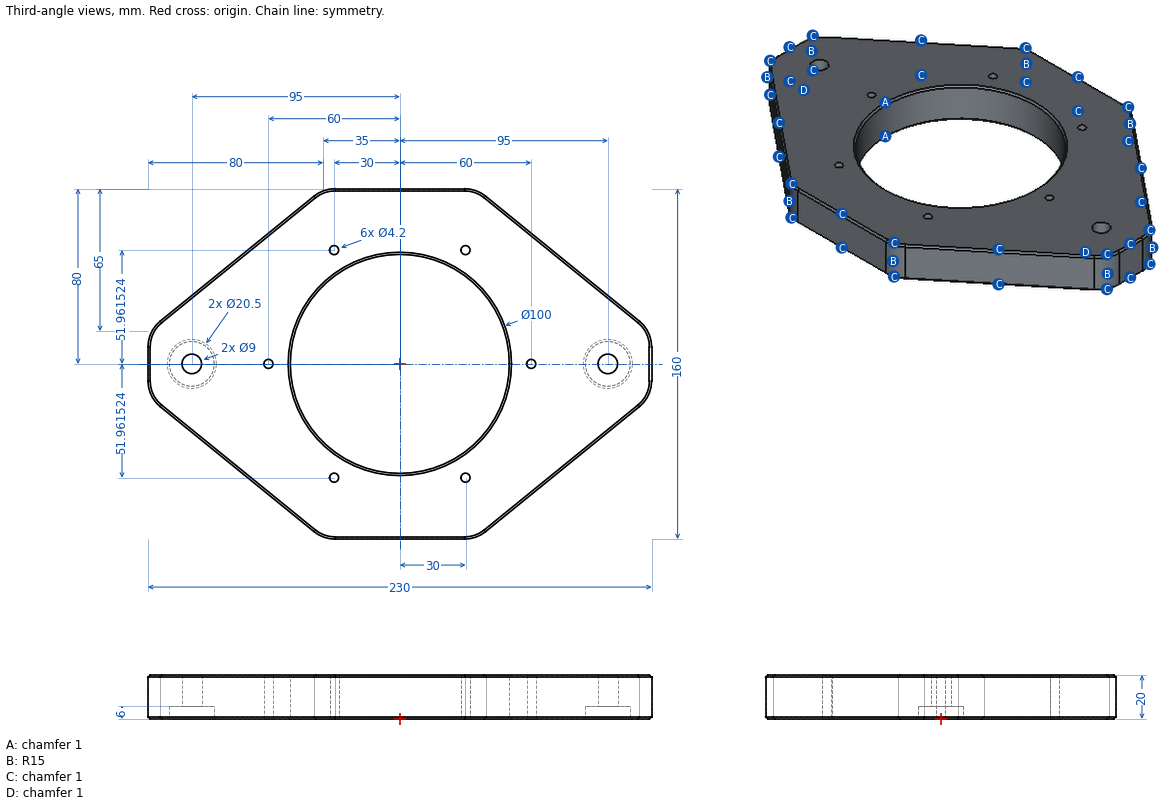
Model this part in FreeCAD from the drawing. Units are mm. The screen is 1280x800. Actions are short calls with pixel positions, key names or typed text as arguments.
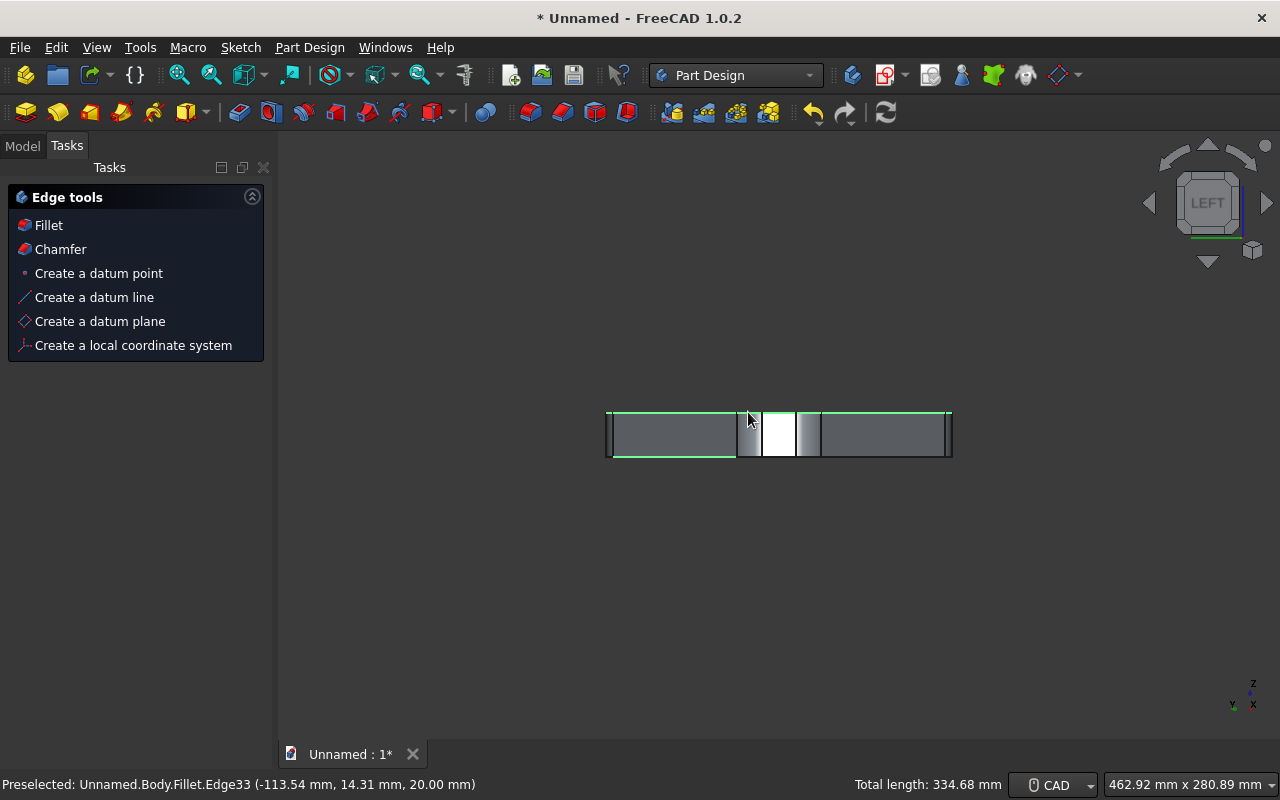
click(779, 456, ctrl)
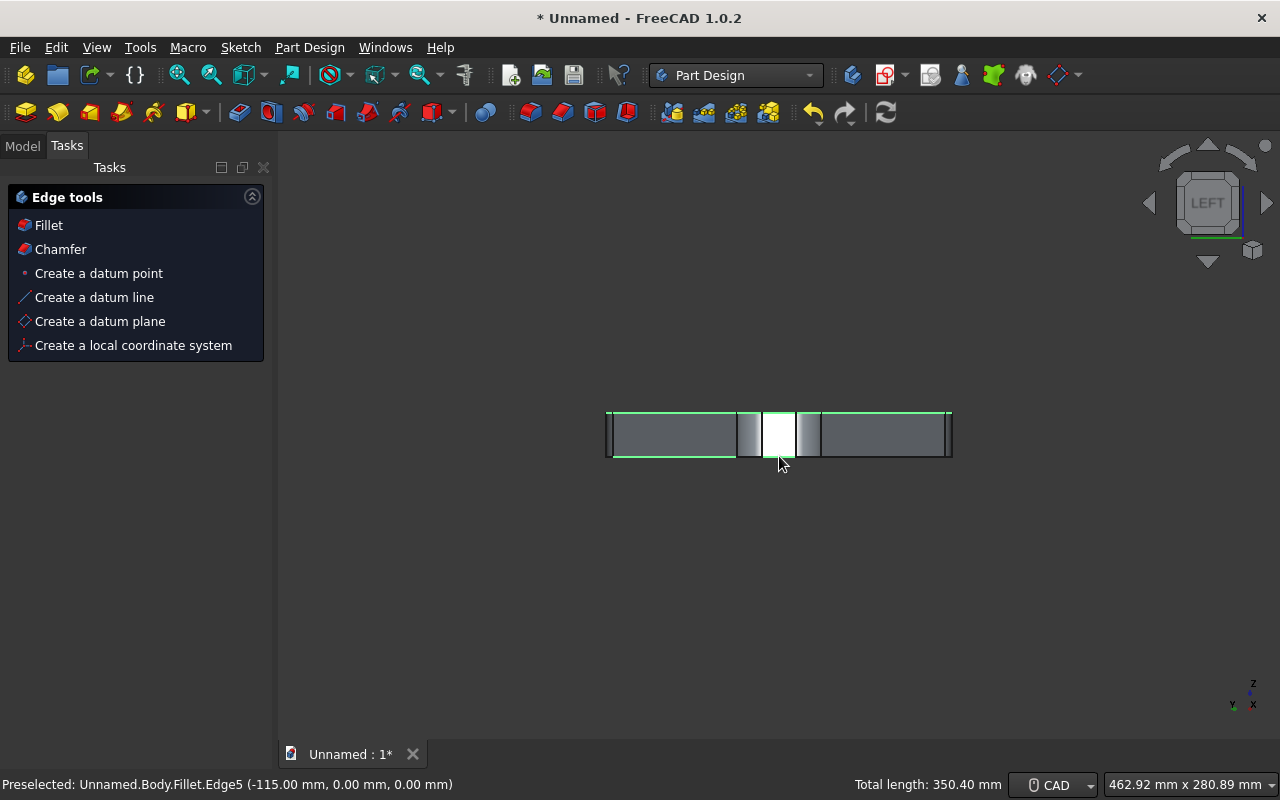
click(883, 456, ctrl)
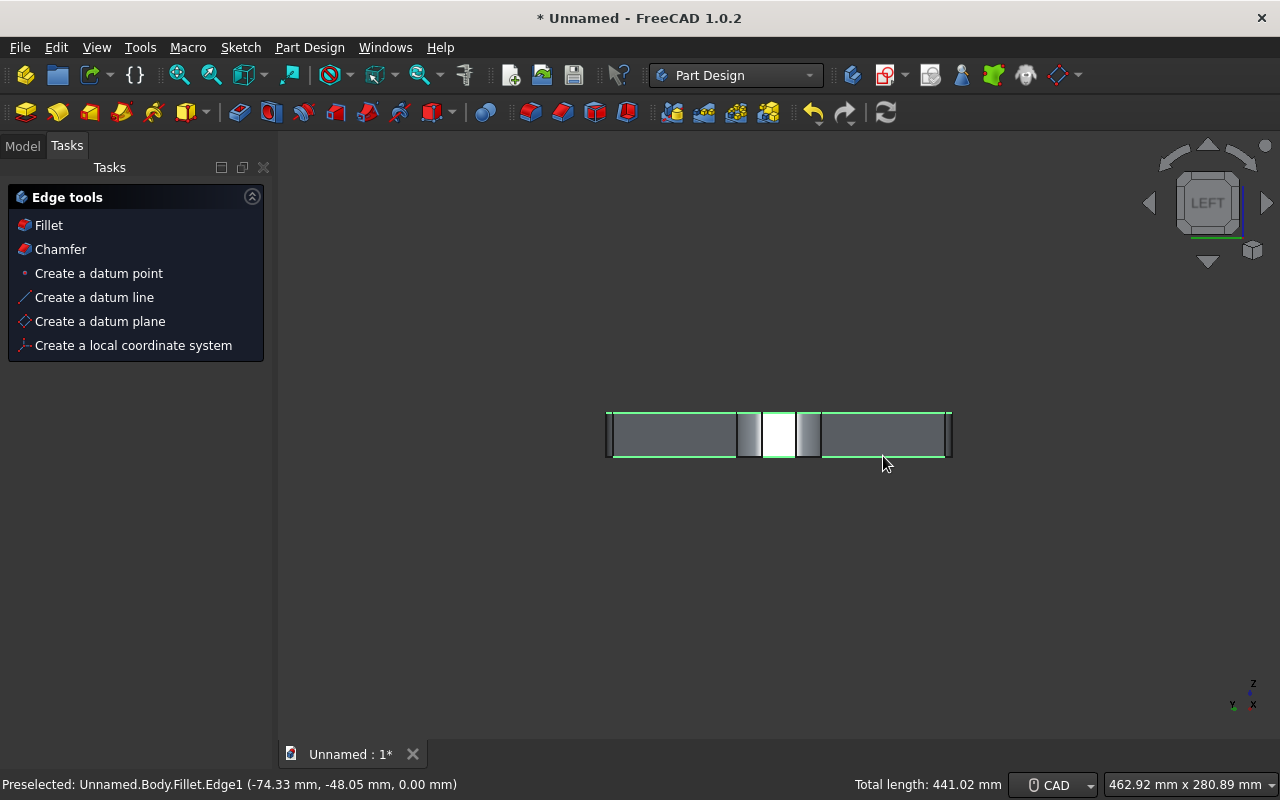
click(810, 456, ctrl)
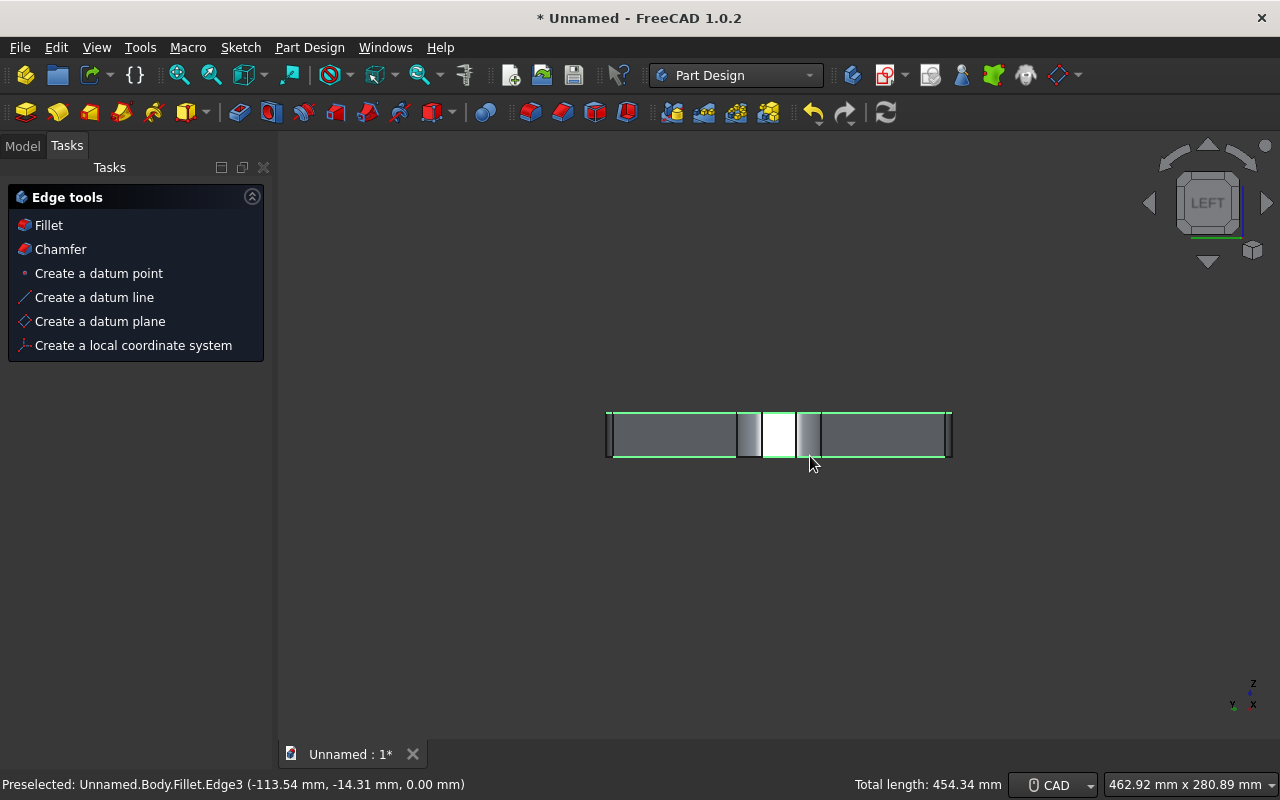
click(951, 456, ctrl)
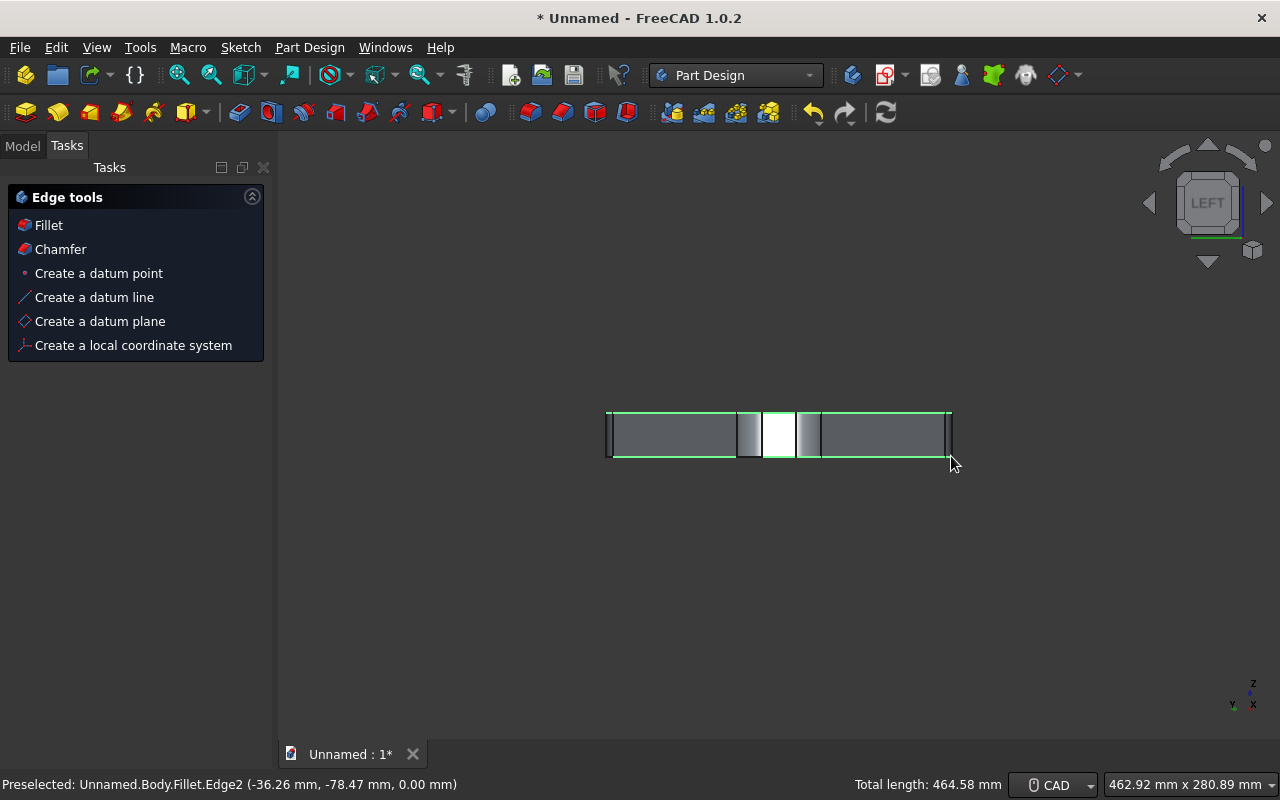
click(607, 456, ctrl)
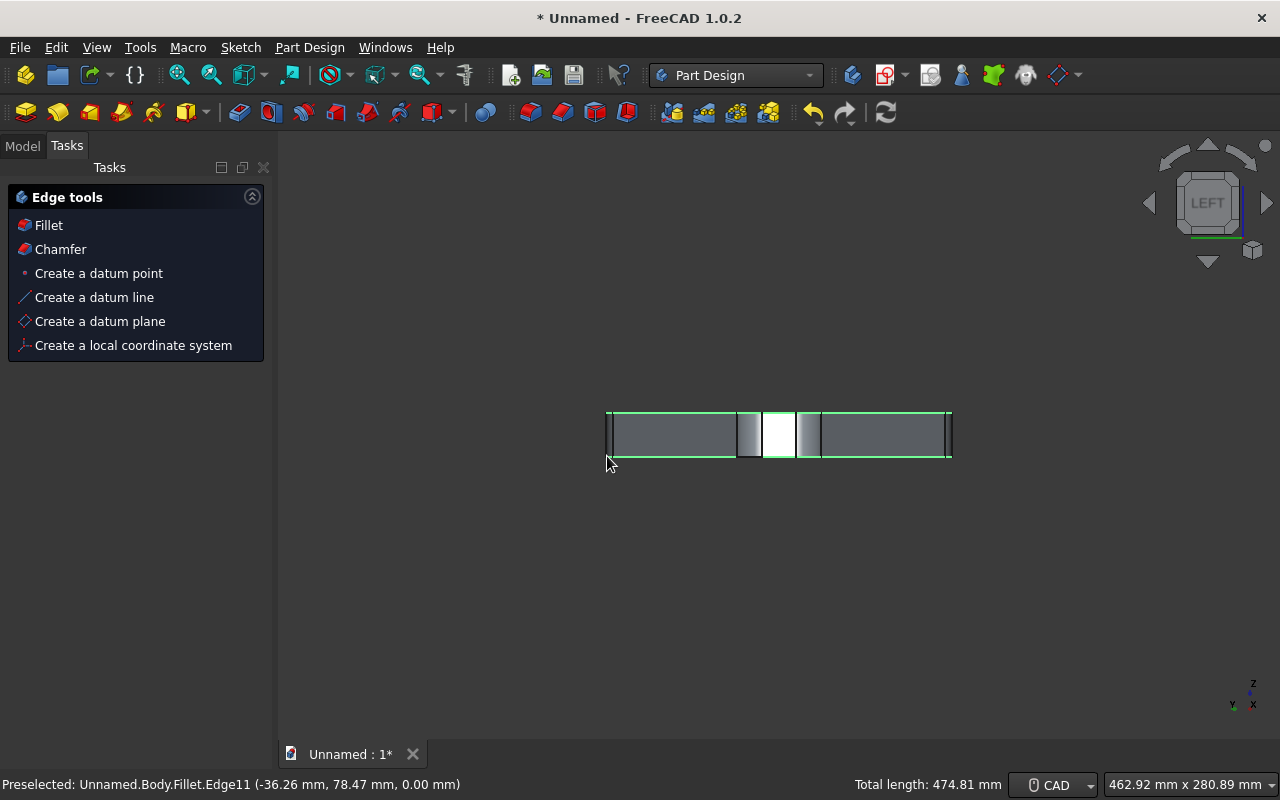
click(748, 456, ctrl)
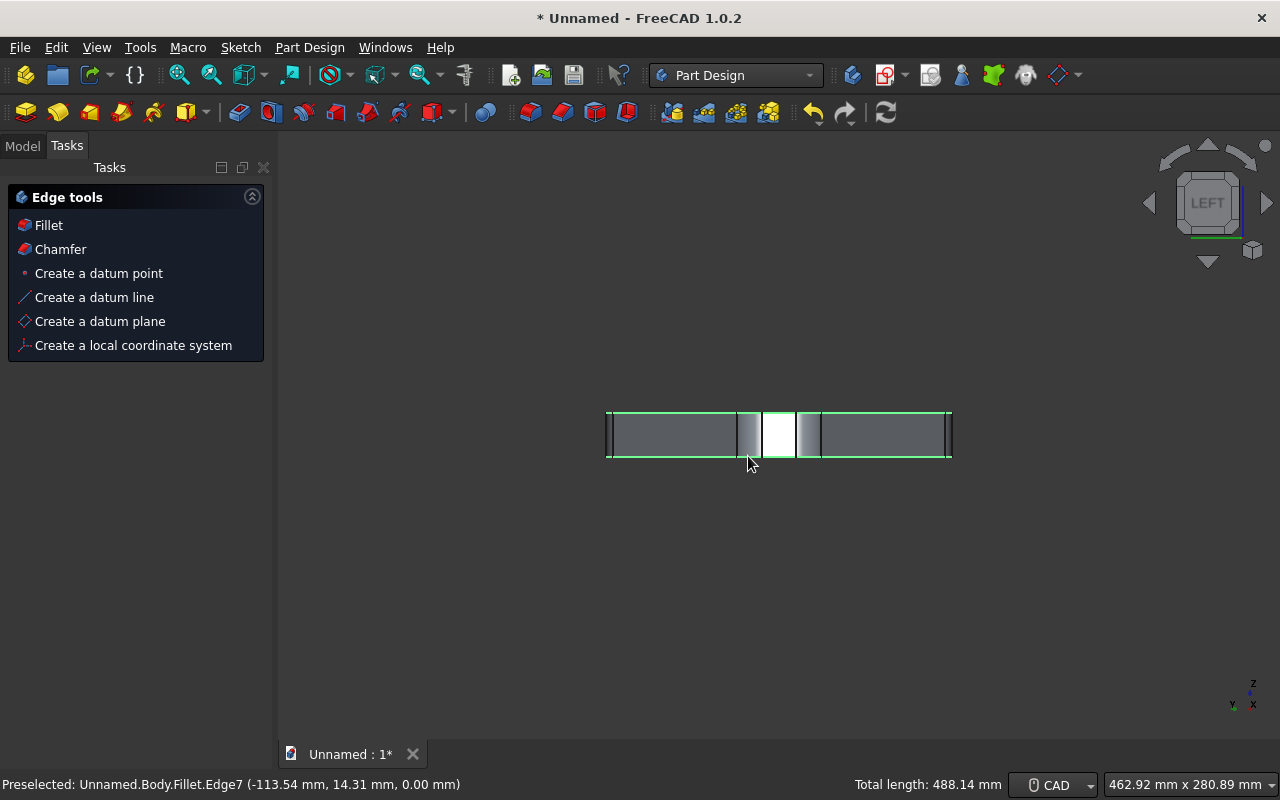
key(0)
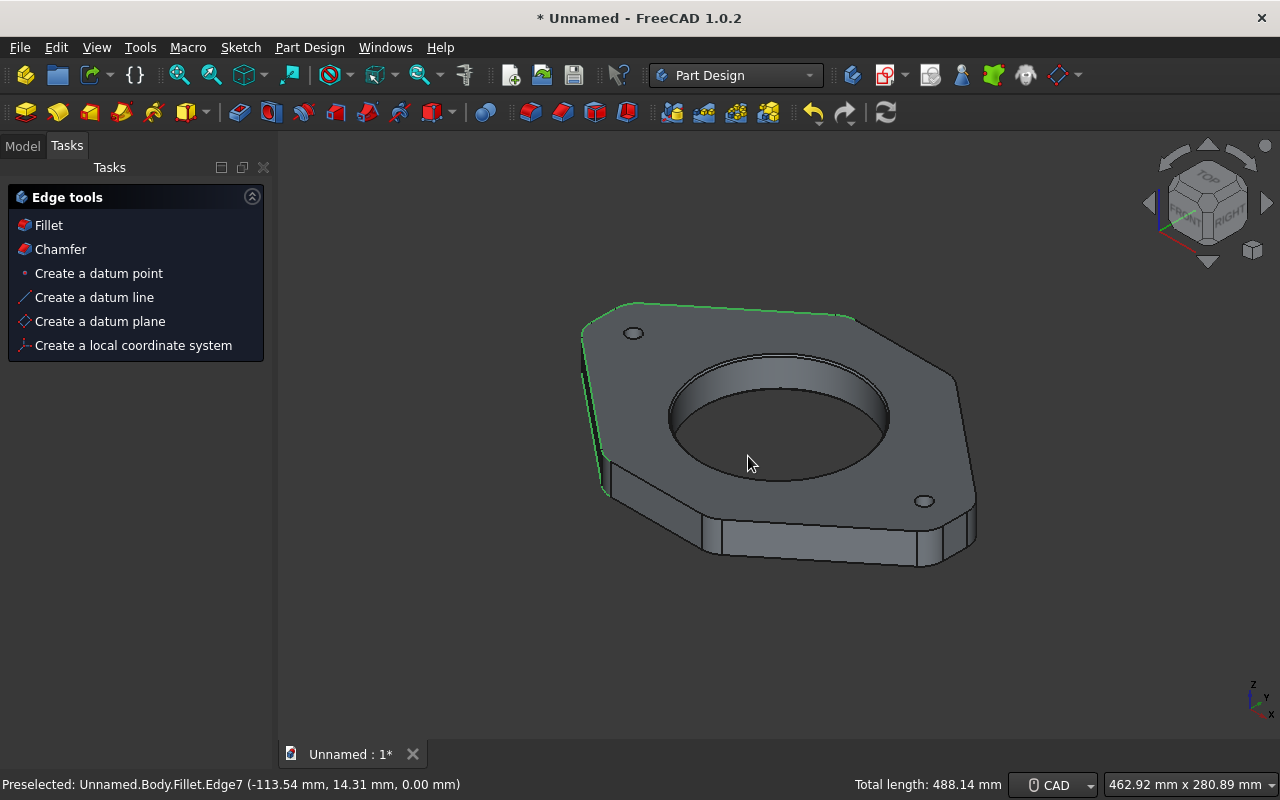
click(955, 518, ctrl)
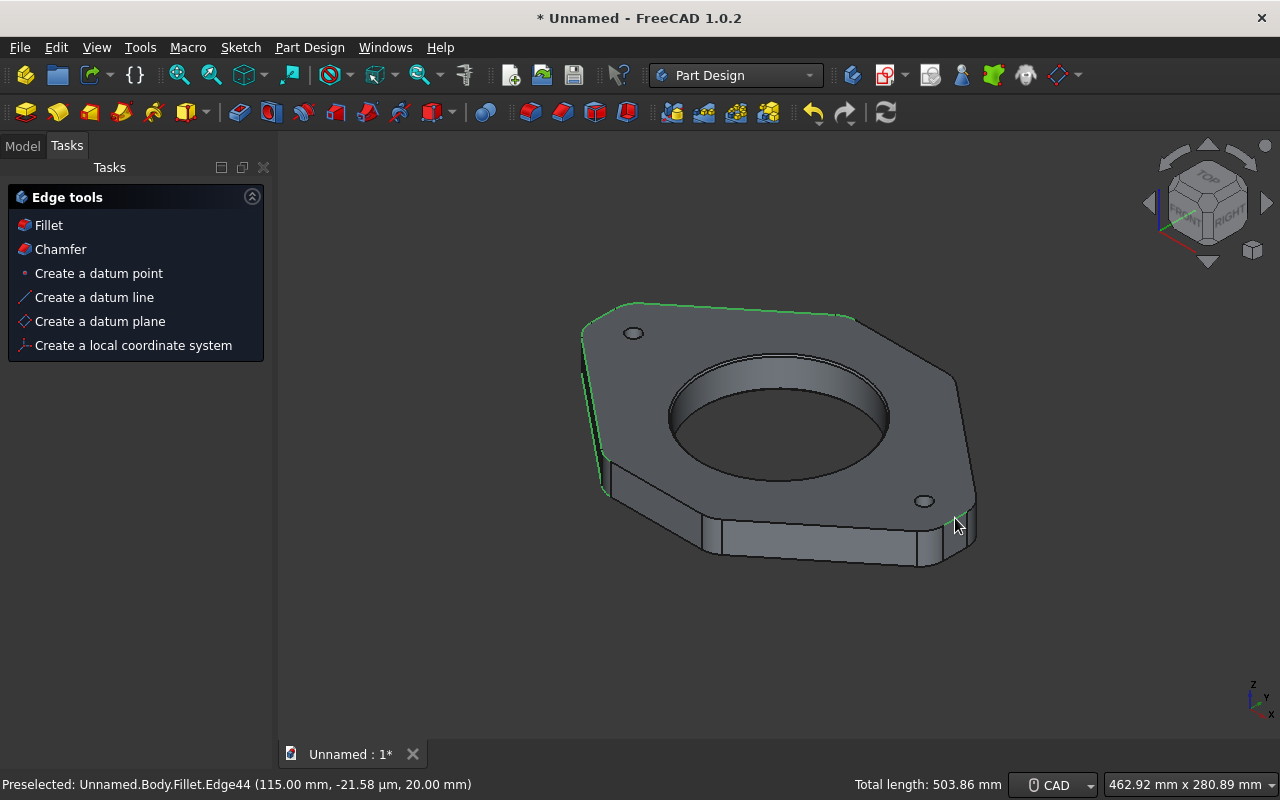
click(657, 487, ctrl)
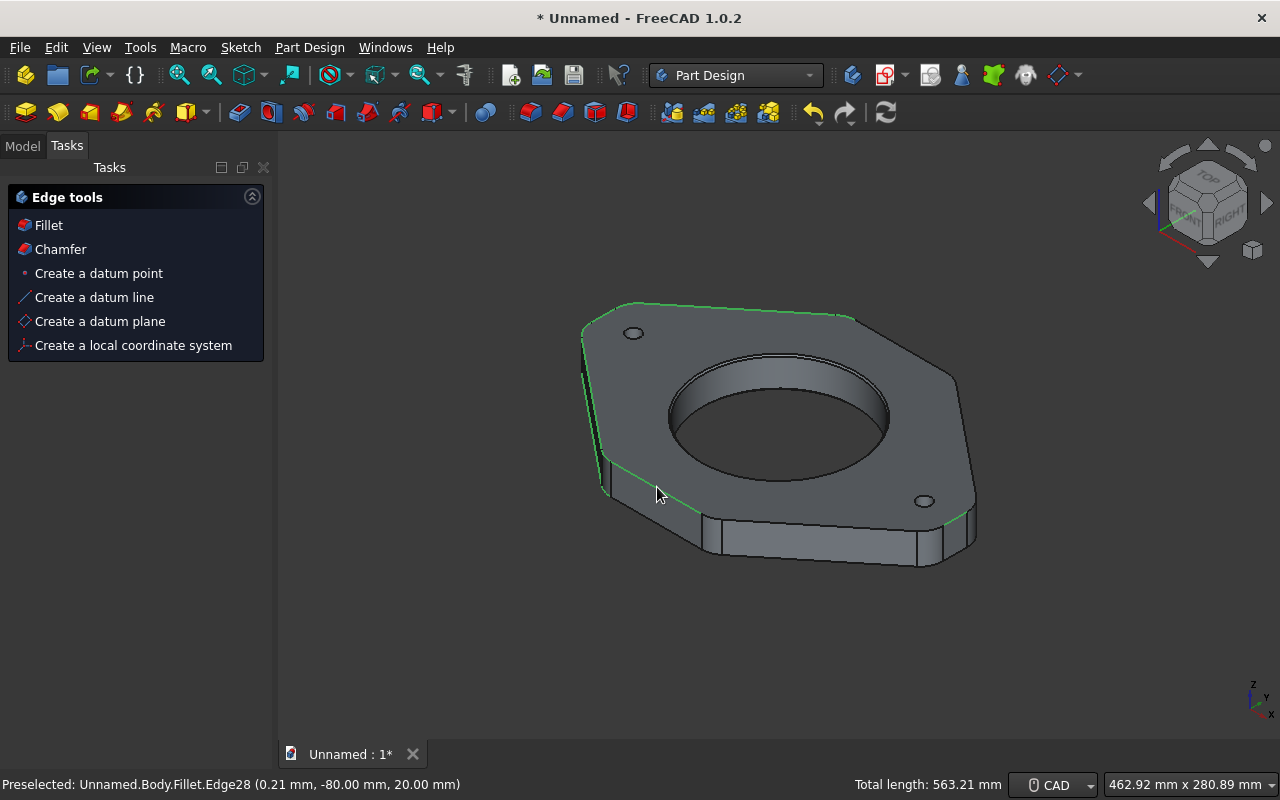
click(819, 524, ctrl)